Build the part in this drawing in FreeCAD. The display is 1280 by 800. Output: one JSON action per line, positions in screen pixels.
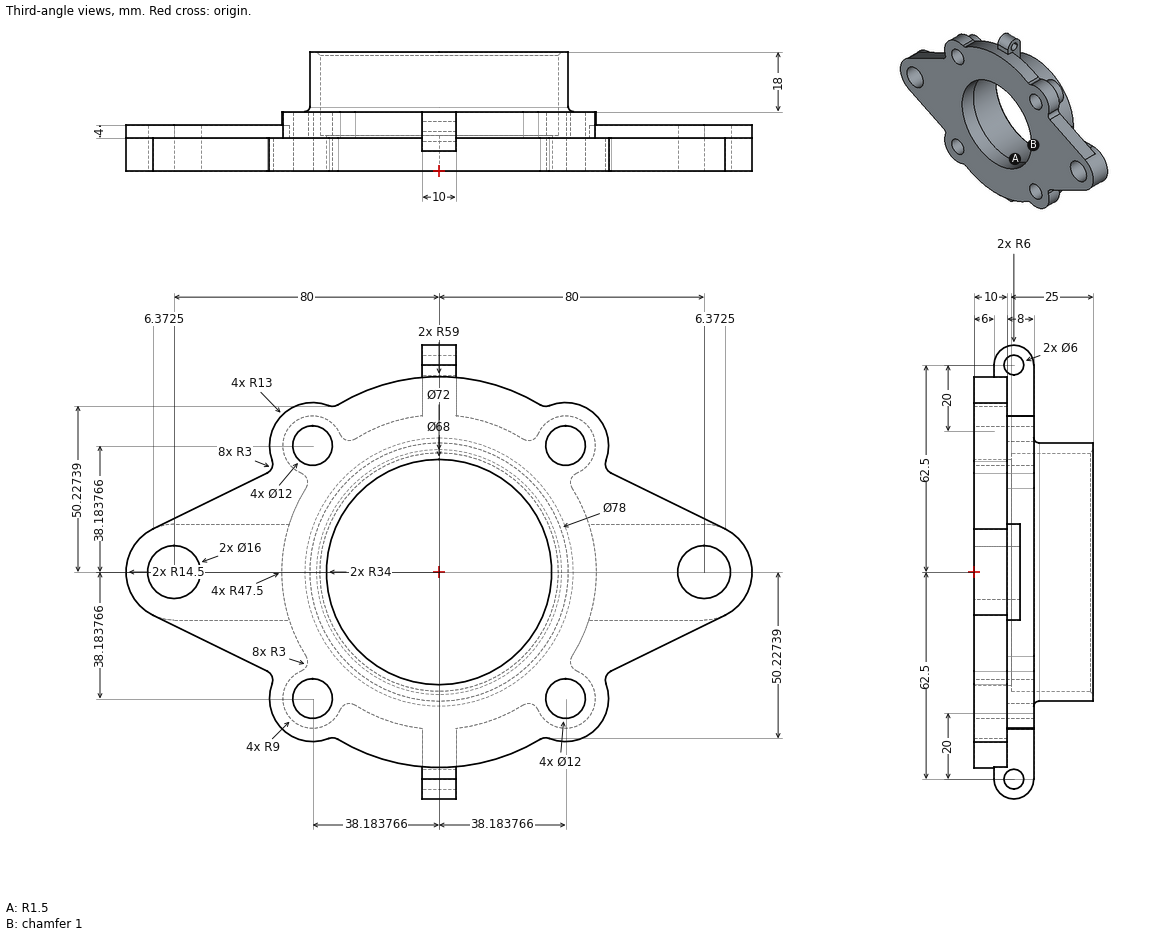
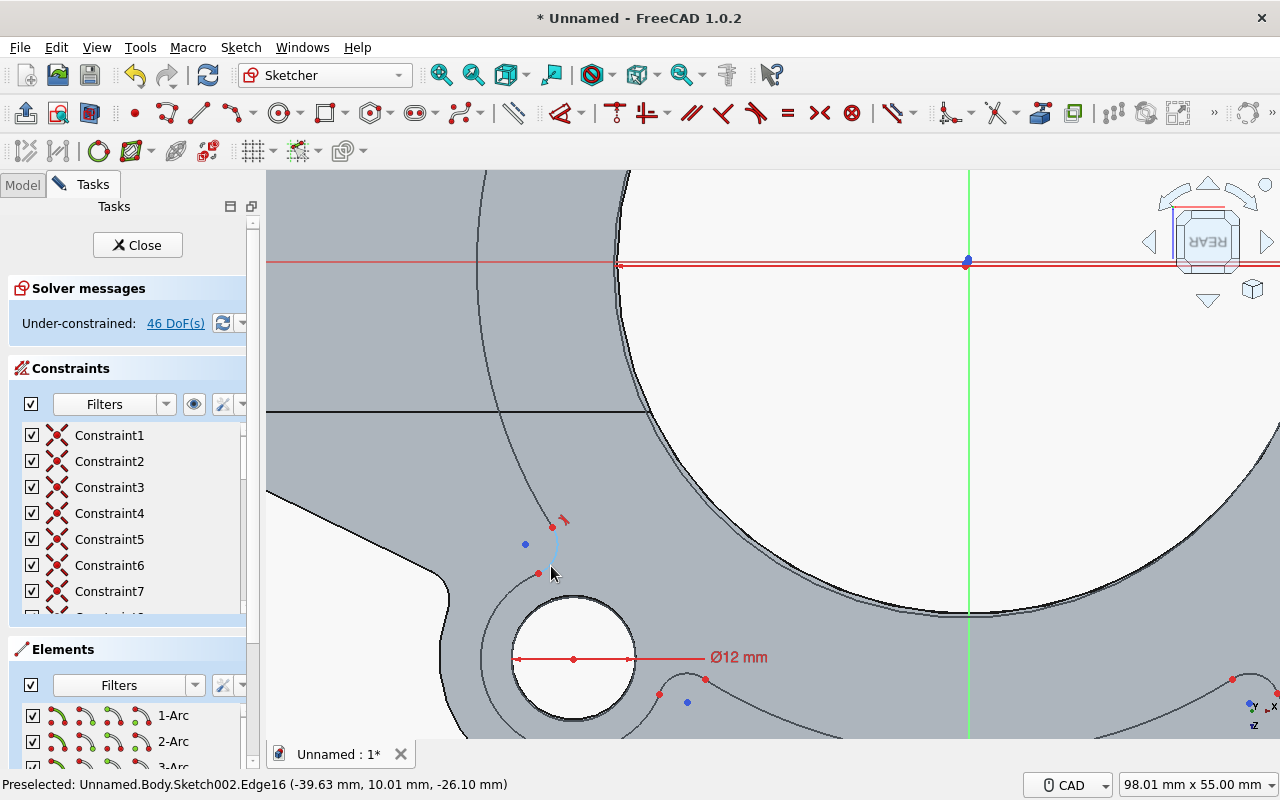
{"action": "left_click", "coordinate": [551, 564]}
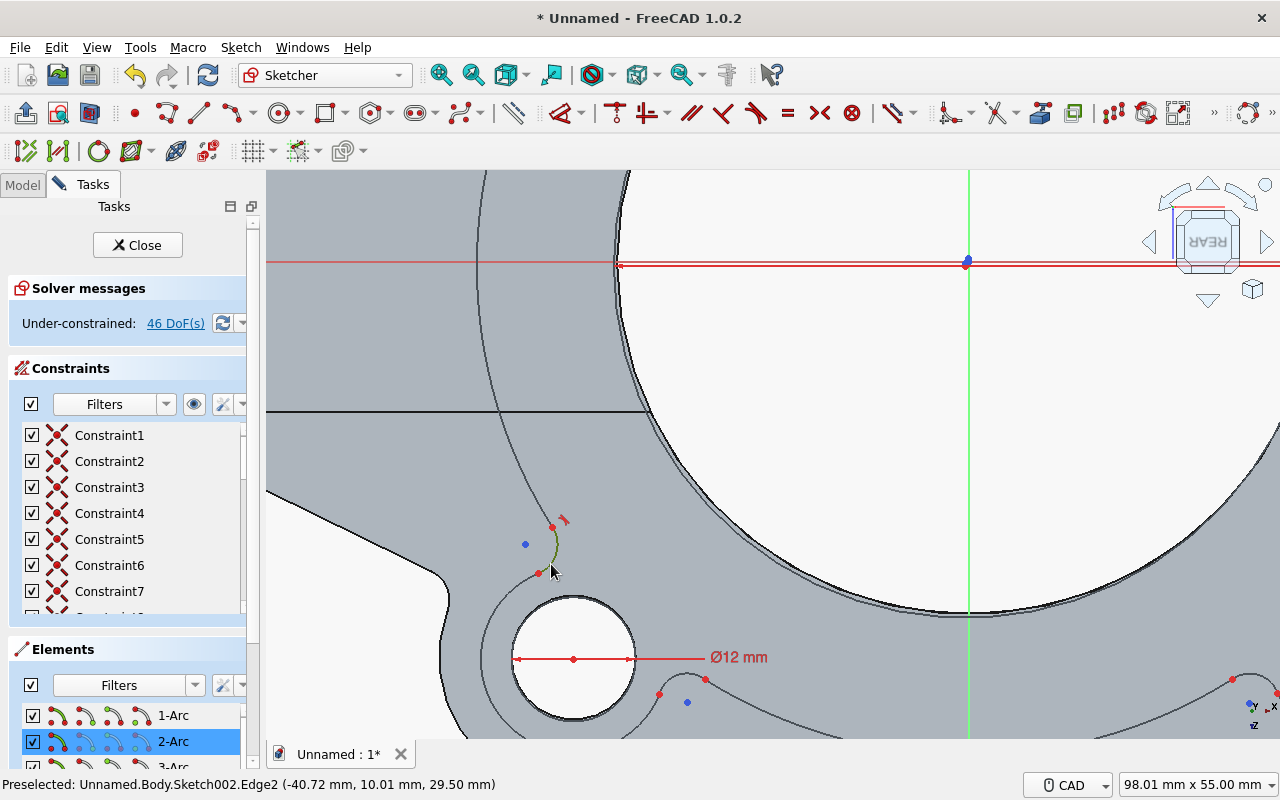
{"action": "left_click", "coordinate": [481, 659]}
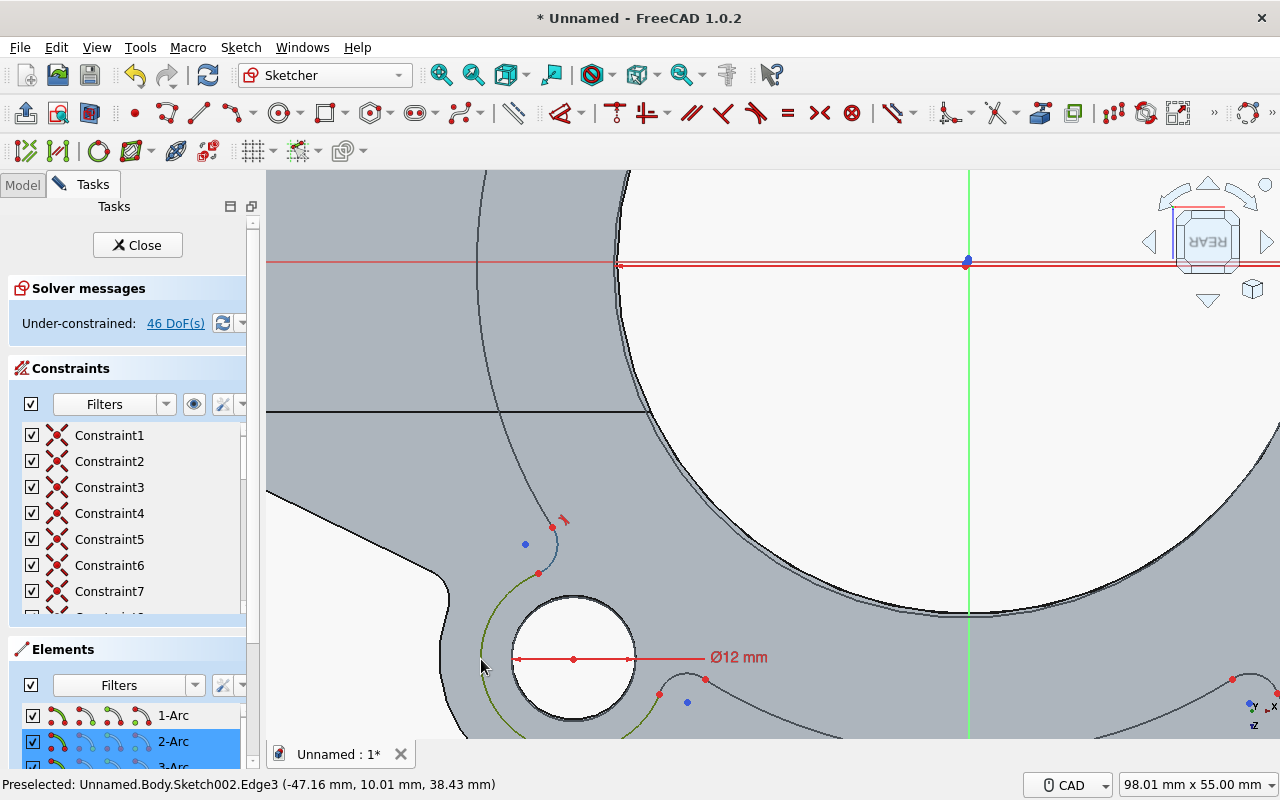
{"action": "left_click", "coordinate": [756, 114]}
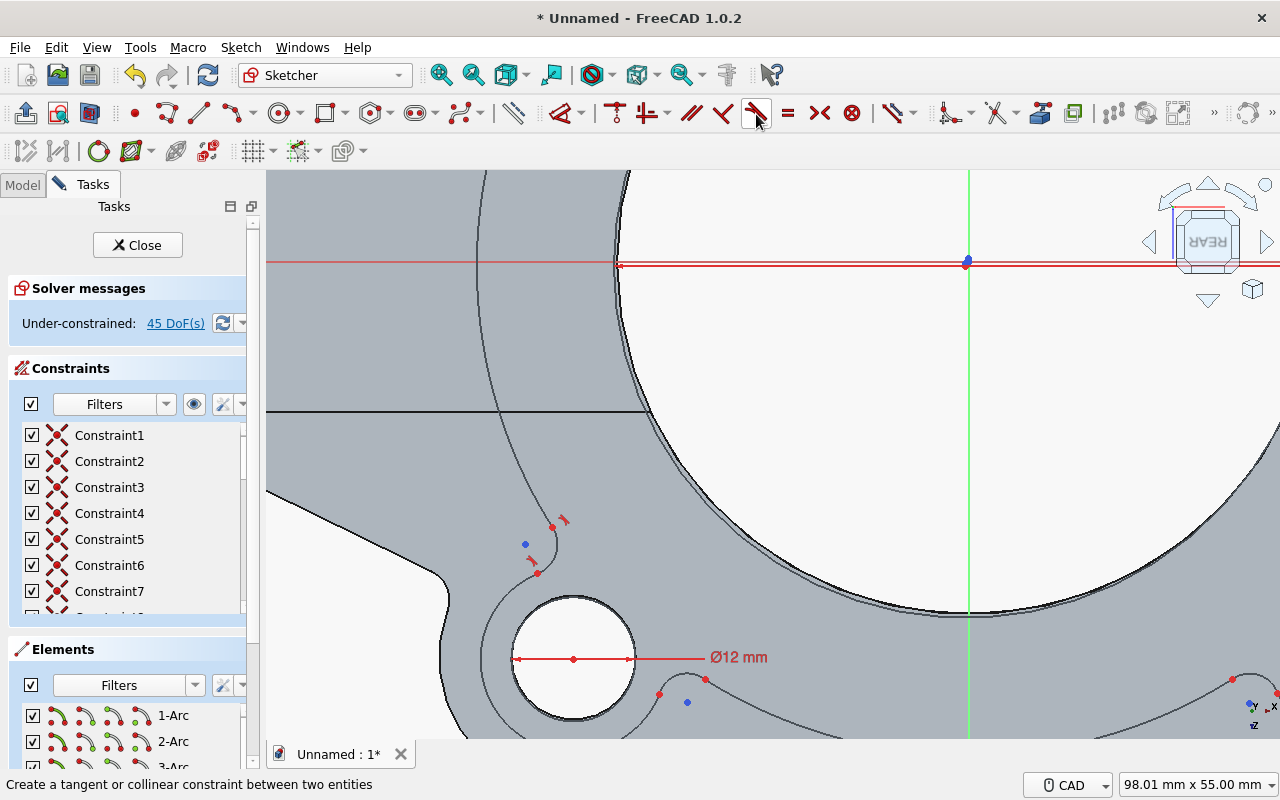
{"action": "left_click", "coordinate": [481, 660]}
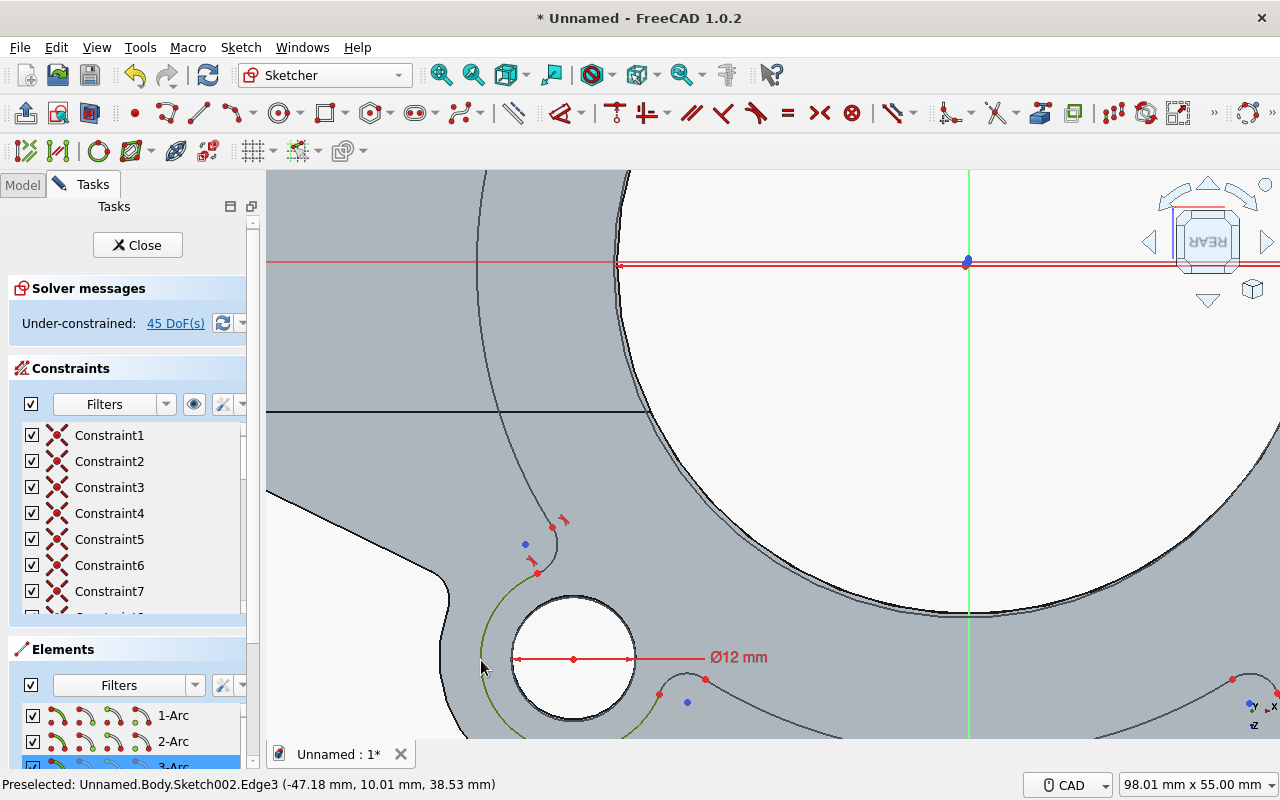
{"action": "left_click", "coordinate": [690, 674]}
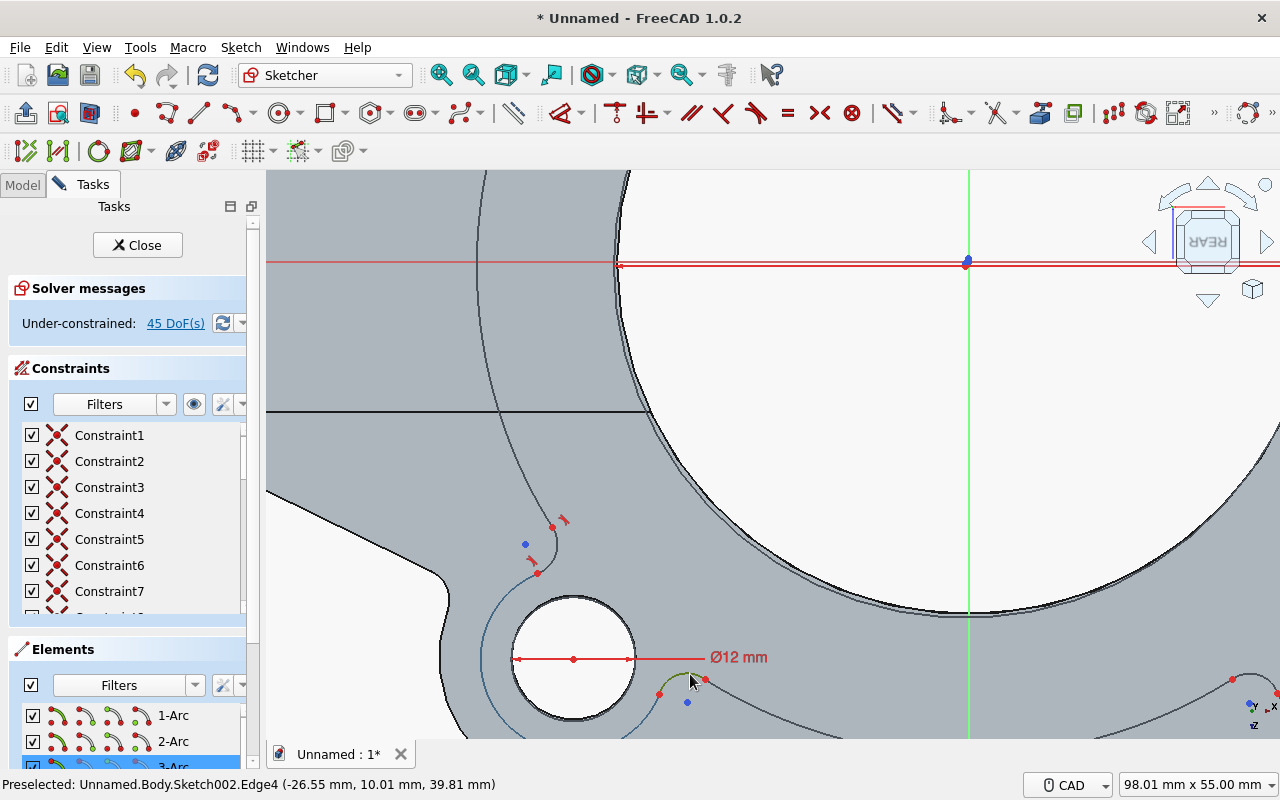
{"action": "left_click", "coordinate": [756, 114]}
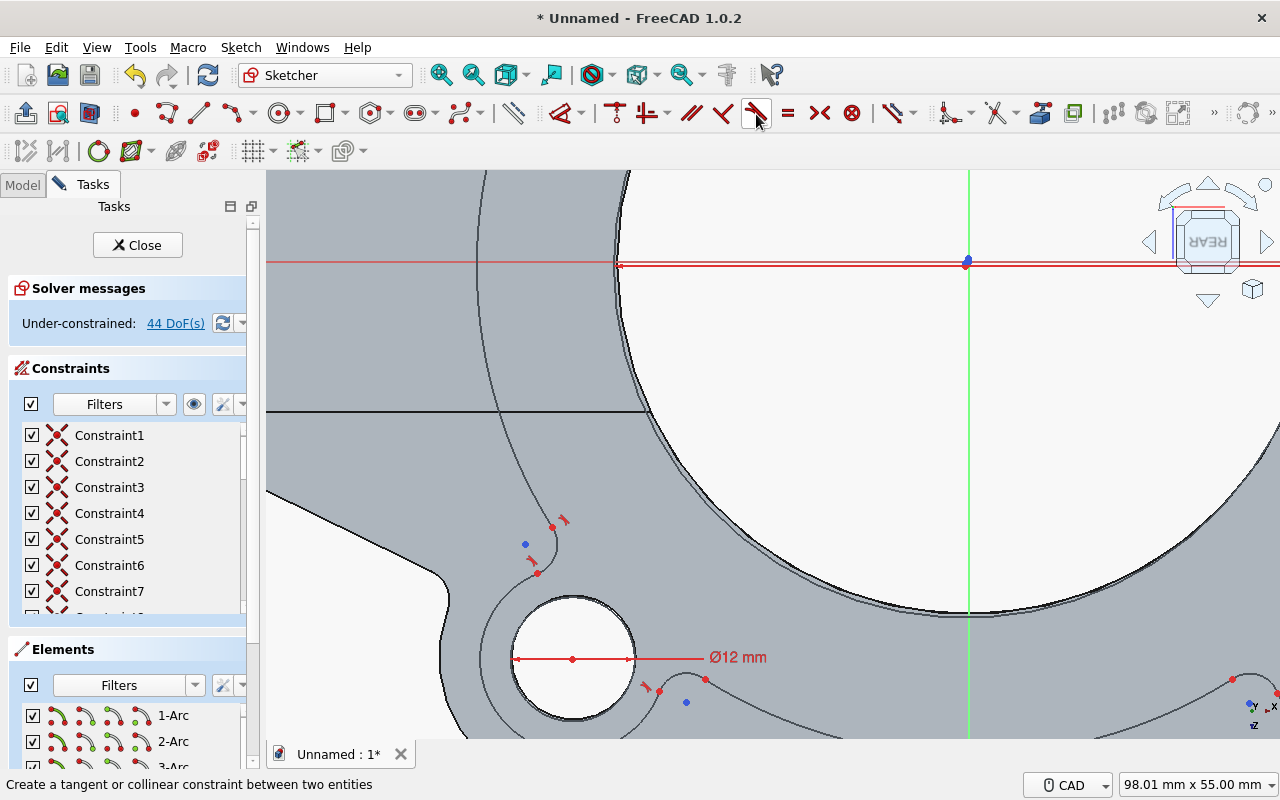
{"action": "left_click", "coordinate": [690, 673]}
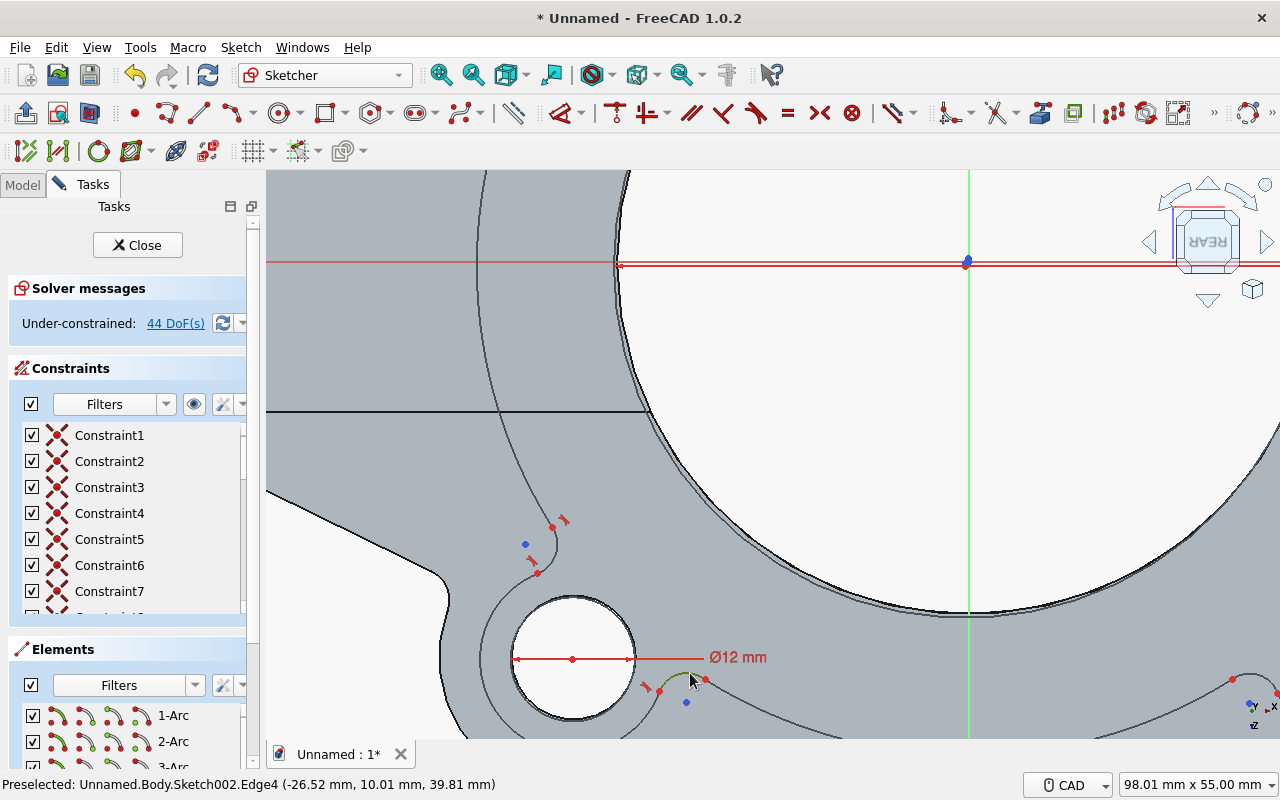
{"action": "scroll", "coordinate": [551, 566], "scroll_direction": "down", "scroll_amount": 5}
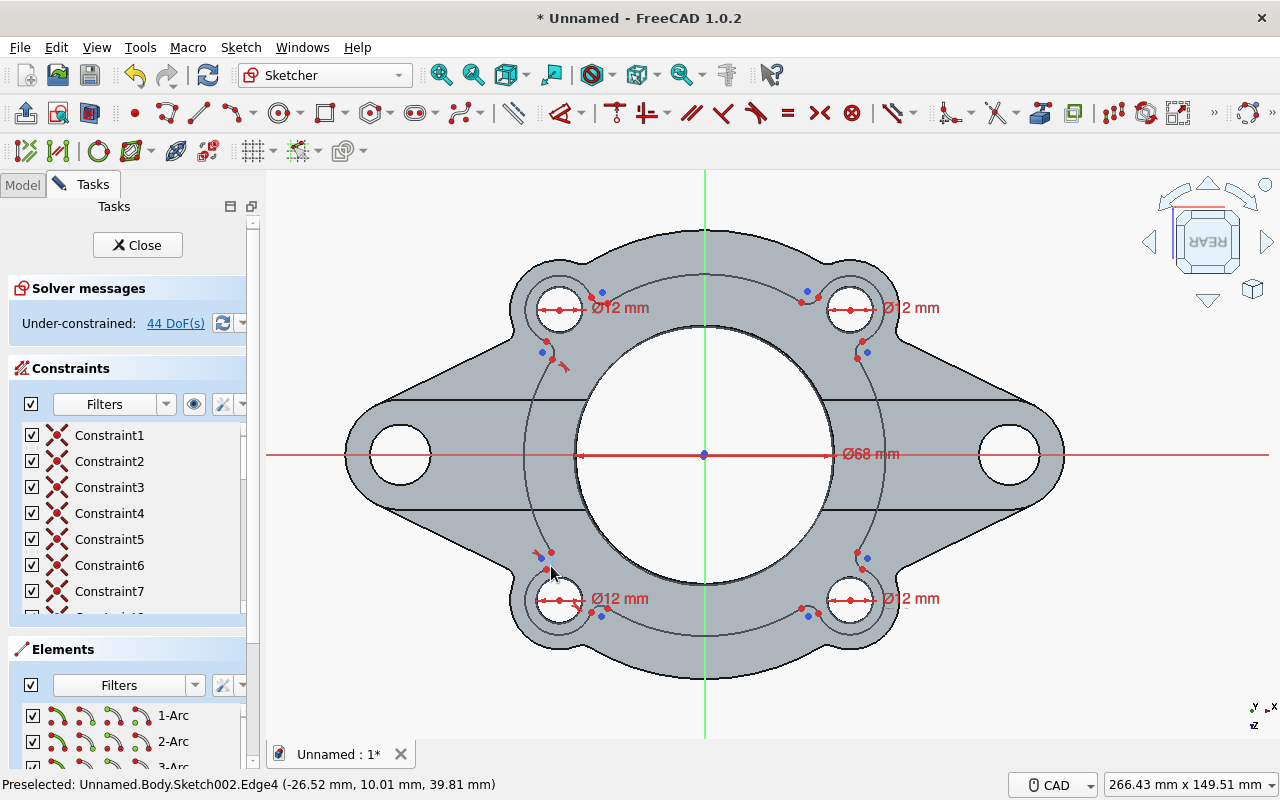
{"action": "left_click", "coordinate": [664, 632]}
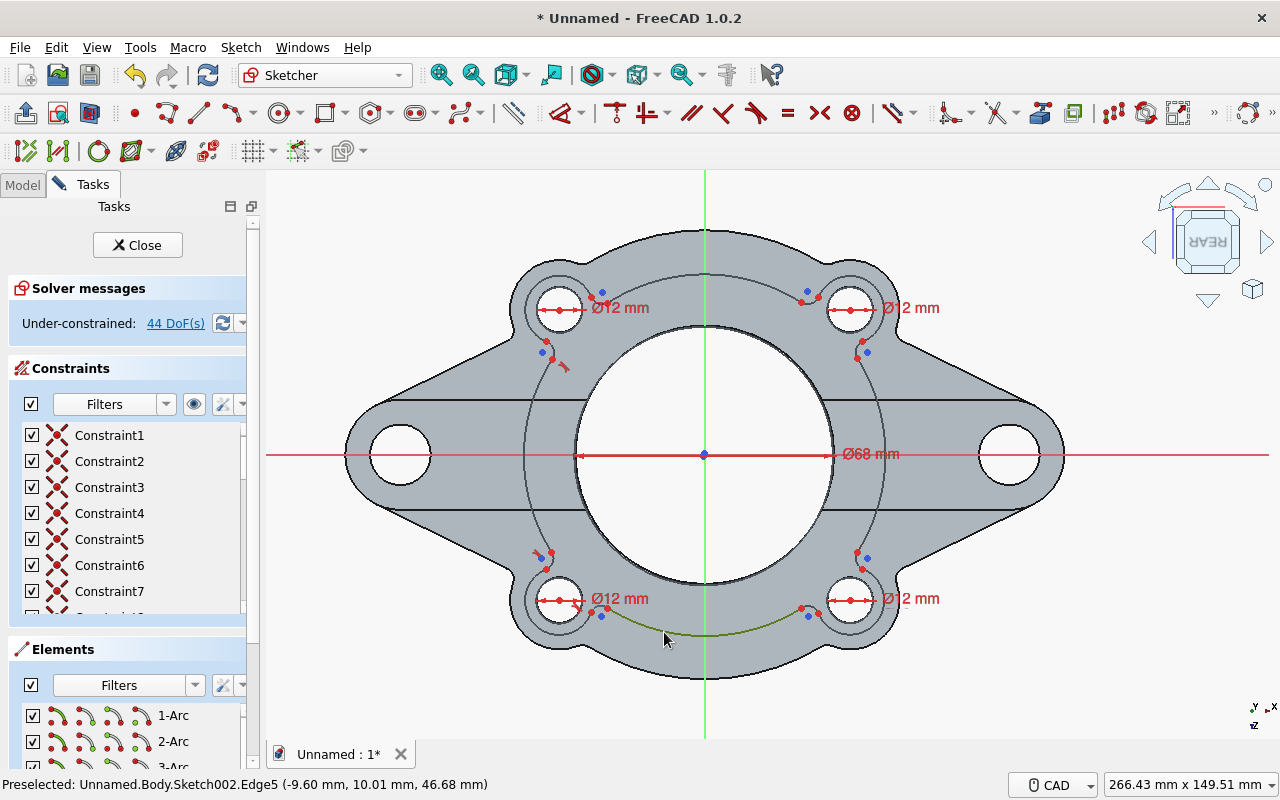
{"action": "left_click", "coordinate": [756, 114]}